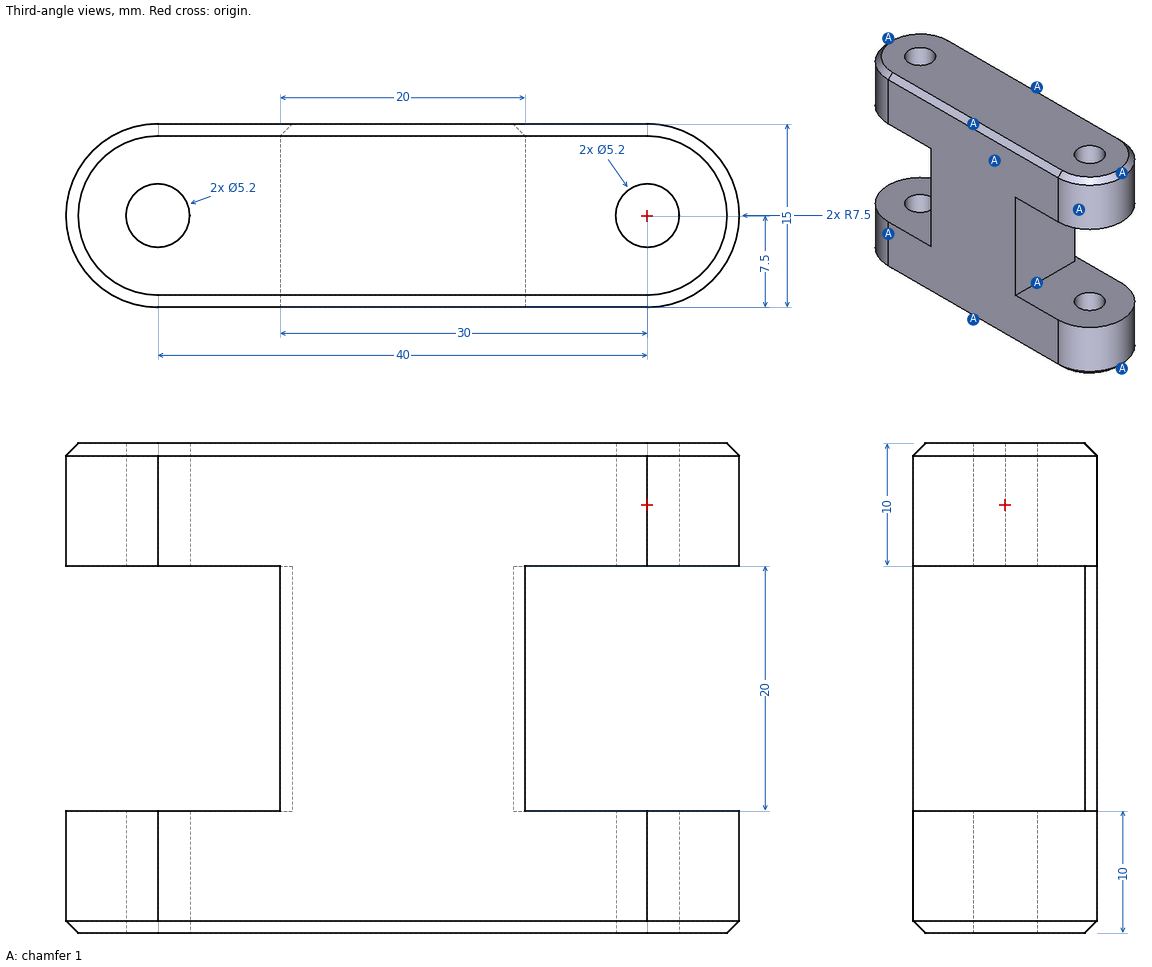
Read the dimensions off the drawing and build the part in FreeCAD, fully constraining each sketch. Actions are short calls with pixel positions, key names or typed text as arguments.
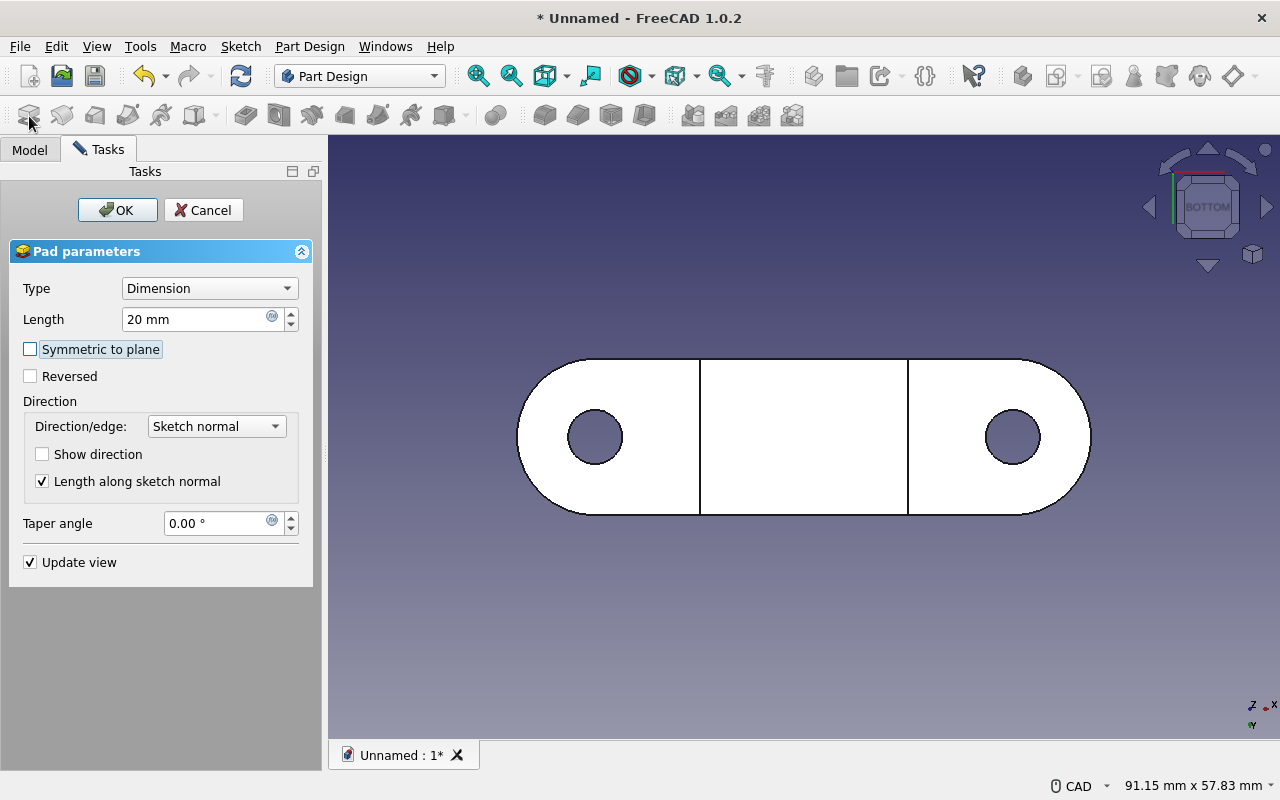
click(118, 210)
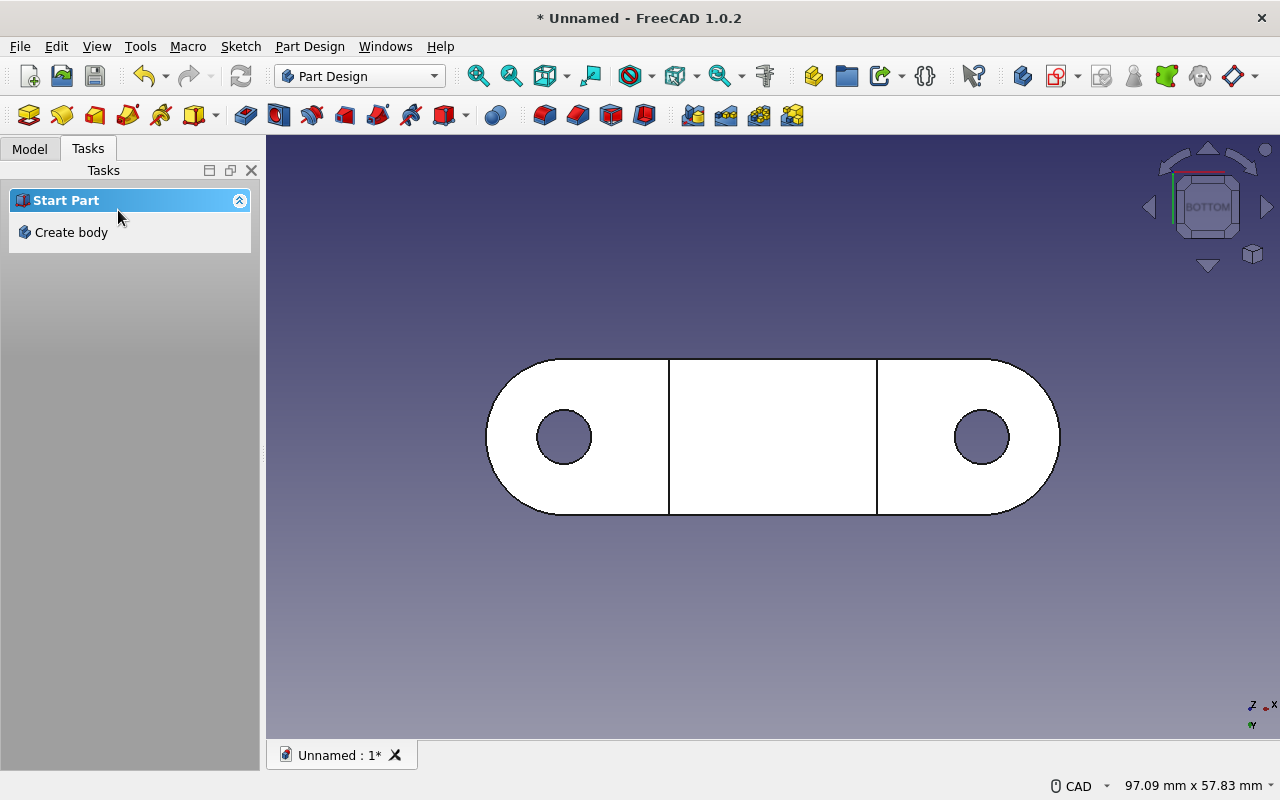
click(773, 436)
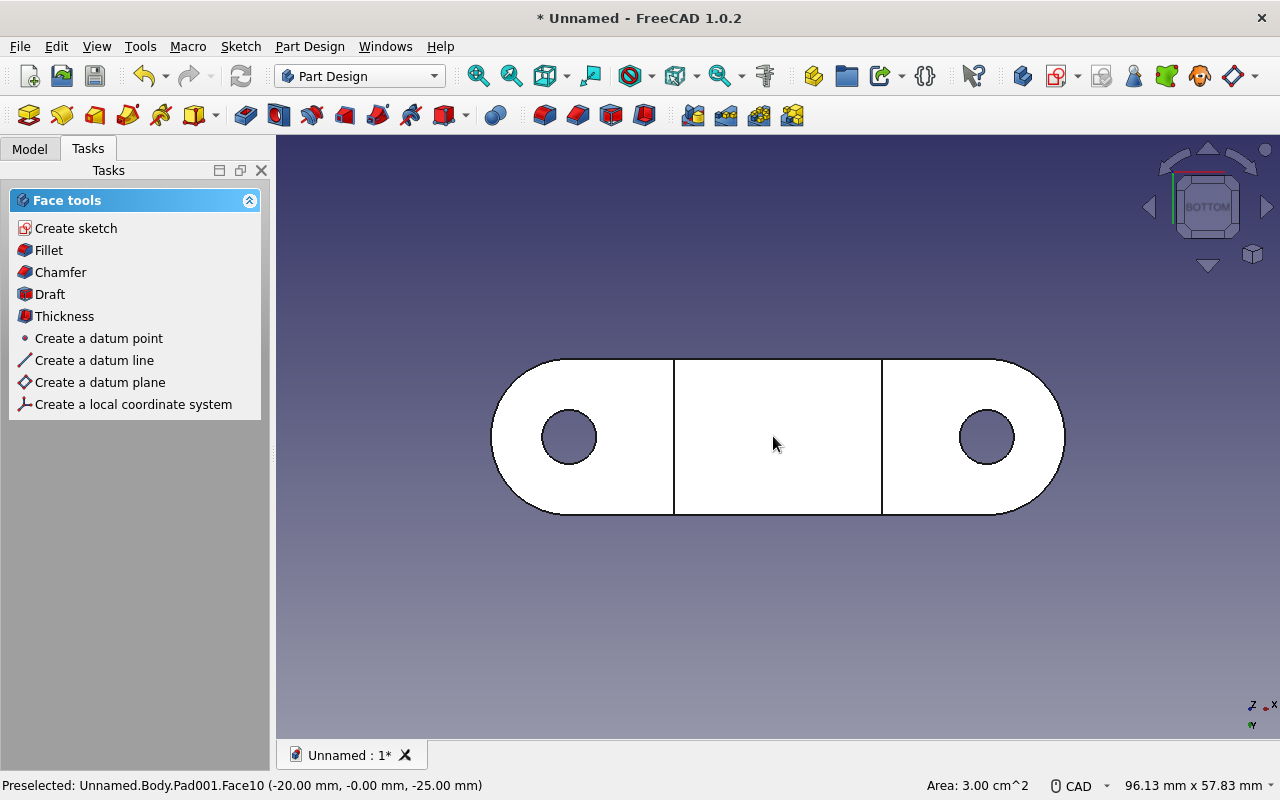
click(1056, 76)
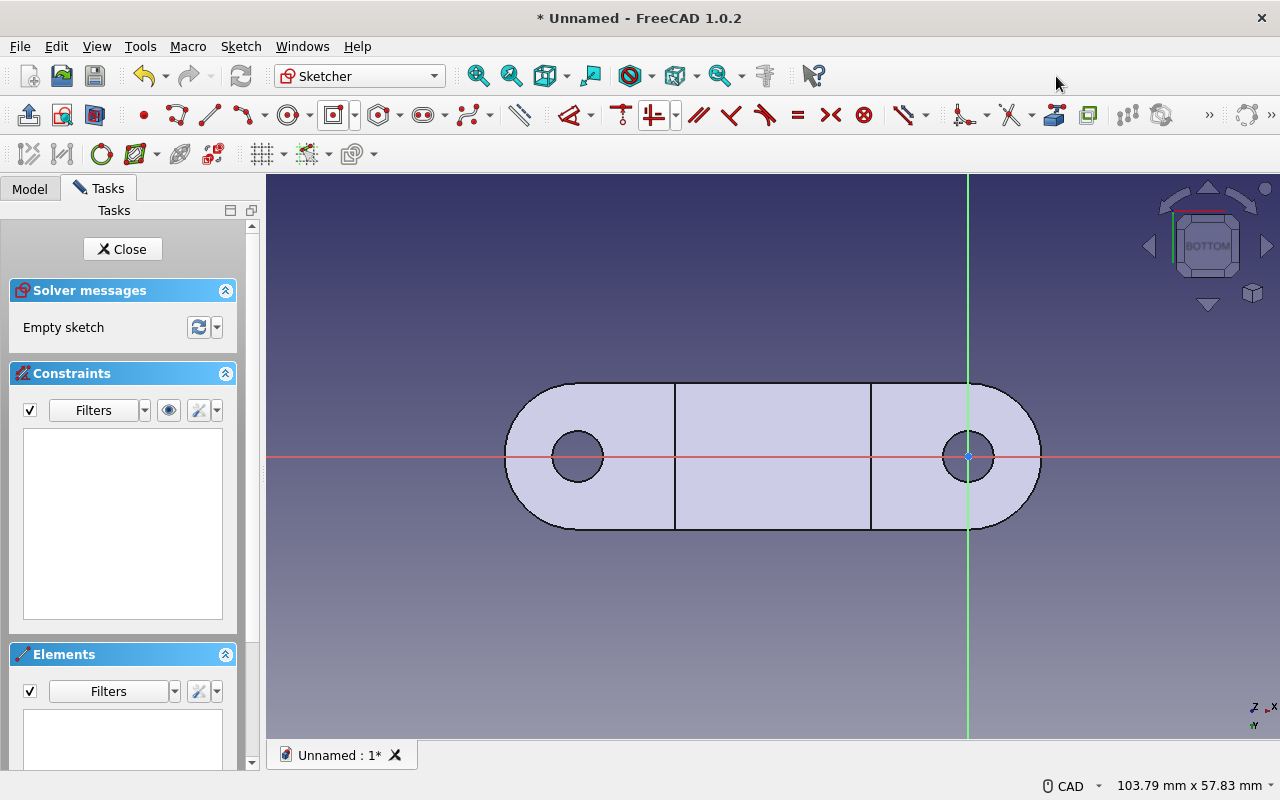
key(g)
key(s)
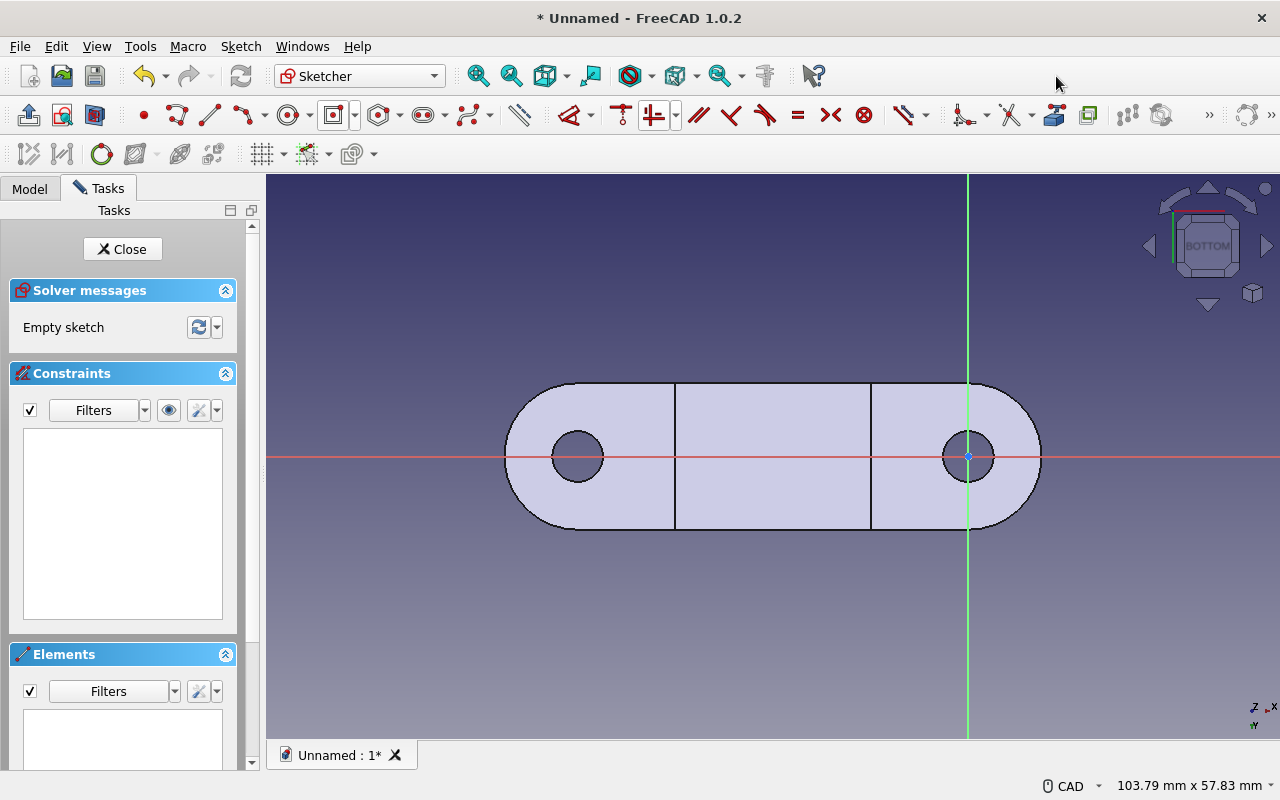
click(968, 457)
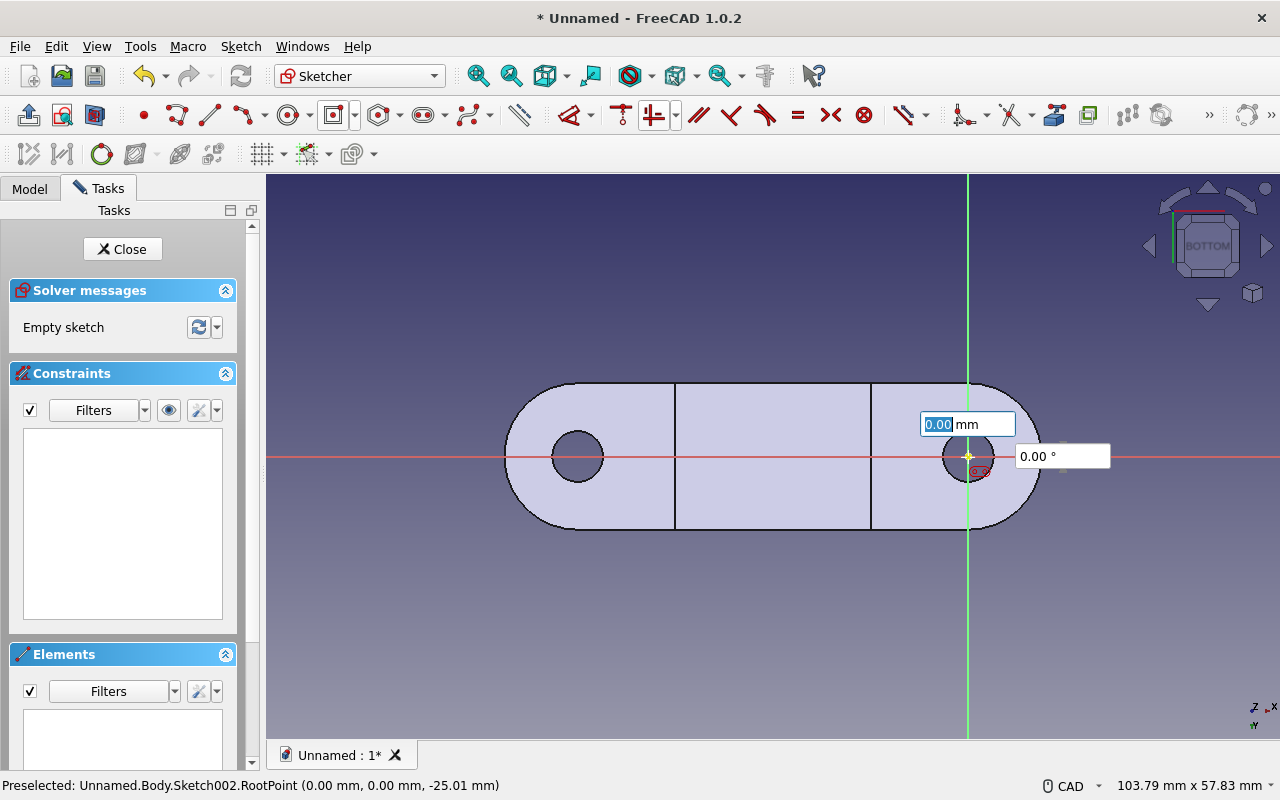
click(578, 448)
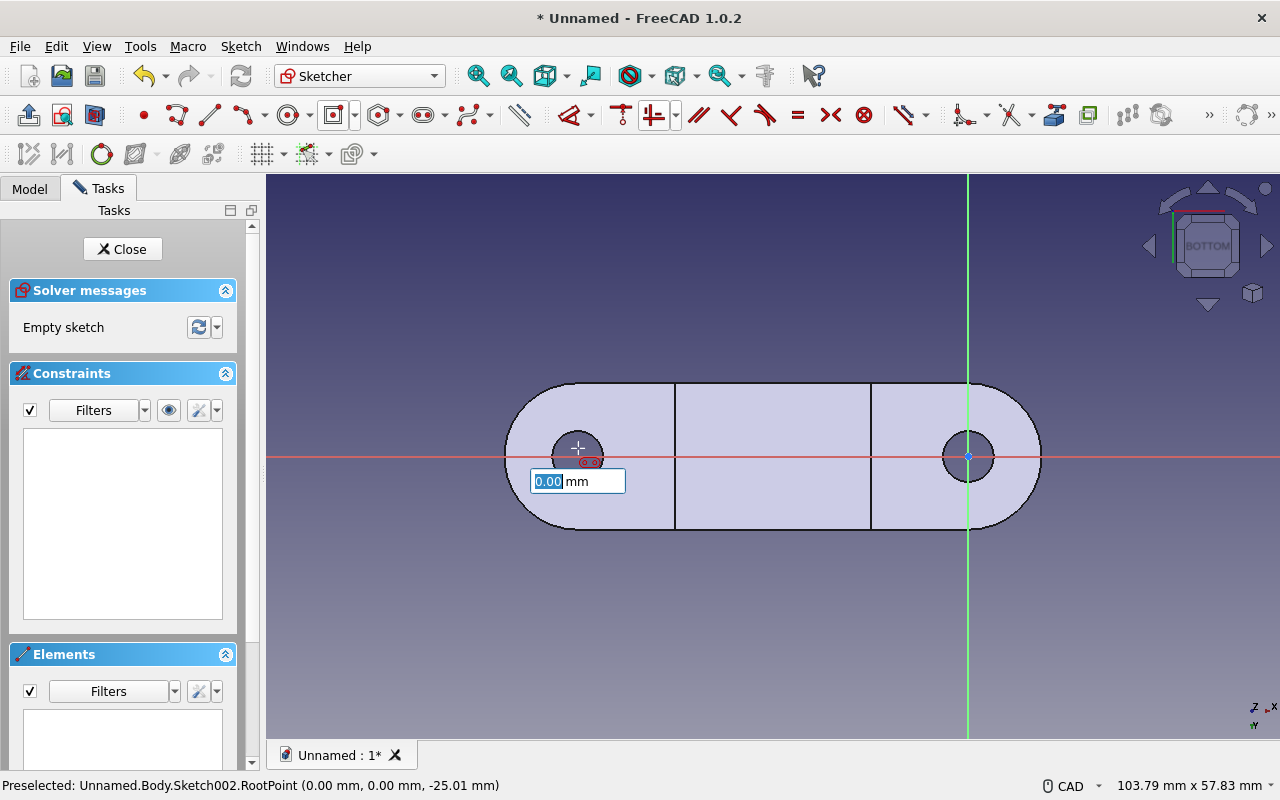
click(773, 530)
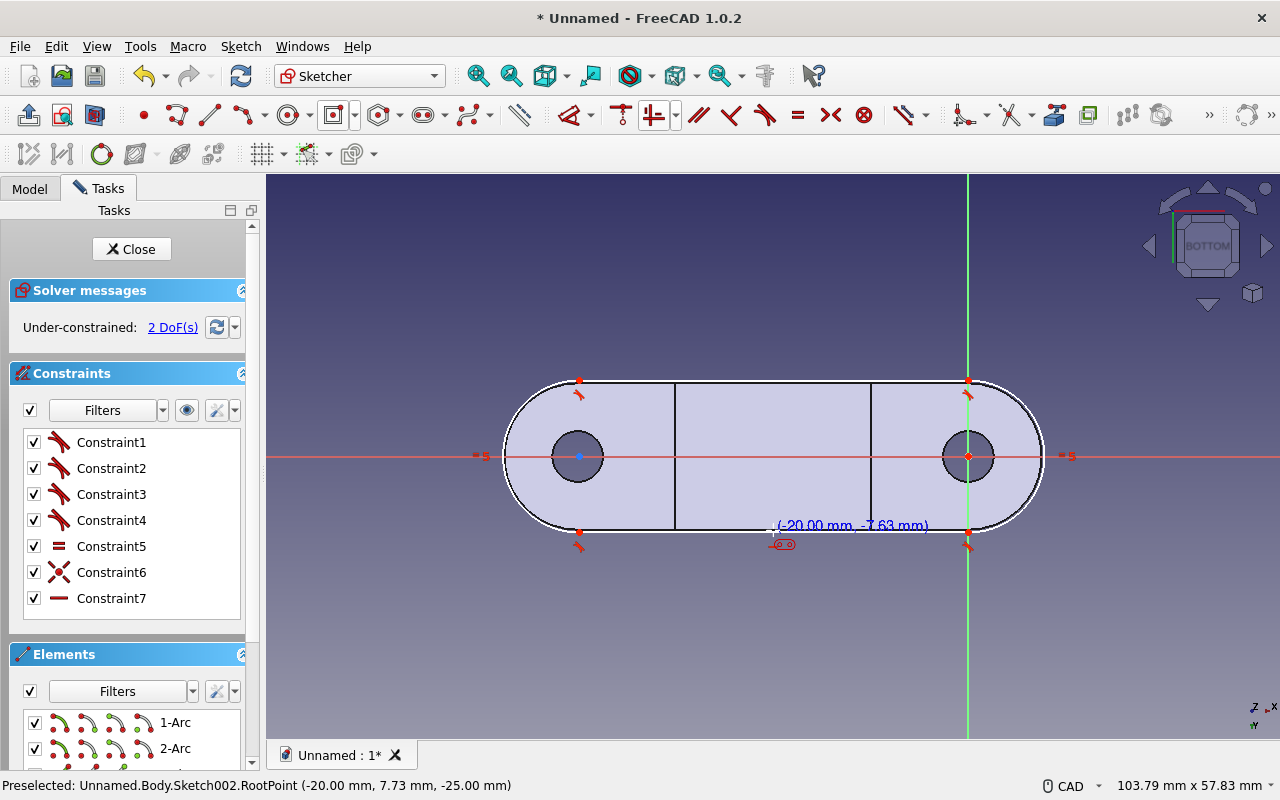
key(g)
key(c)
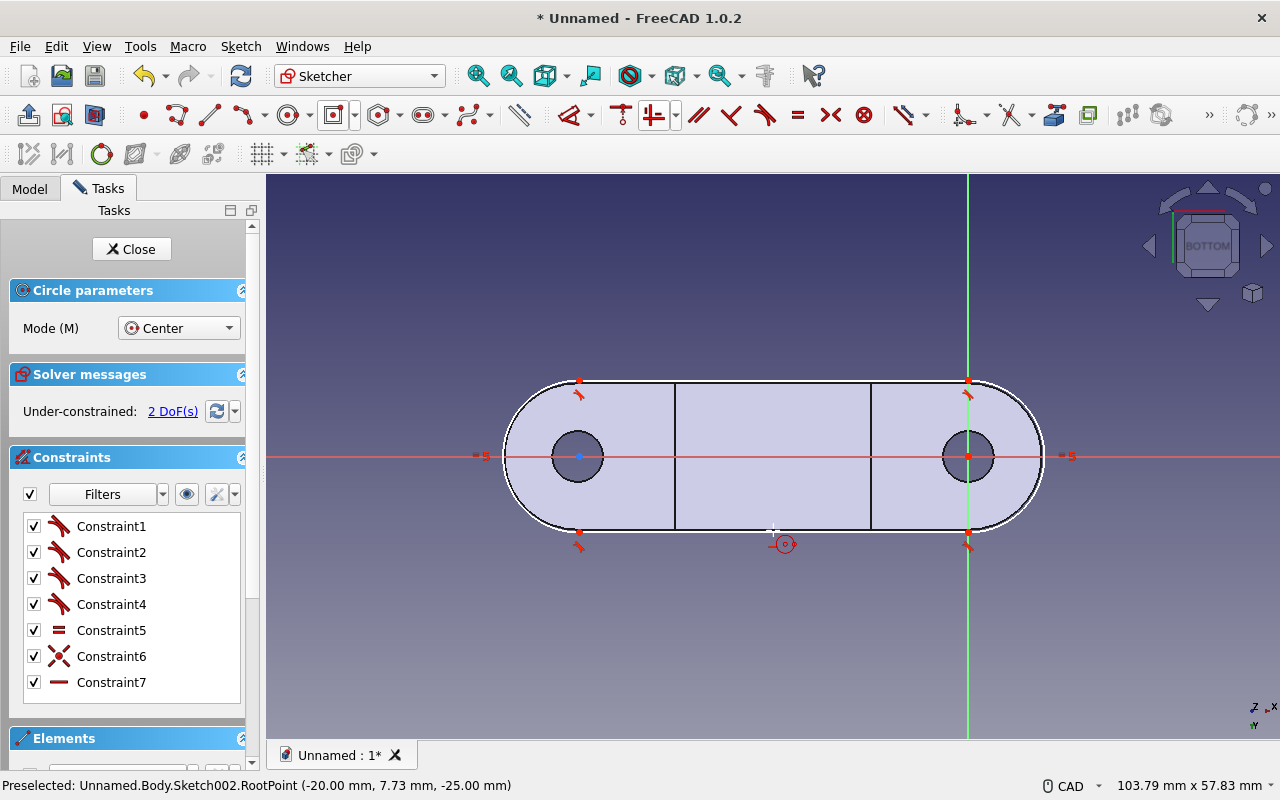
click(579, 457)
move(596, 439)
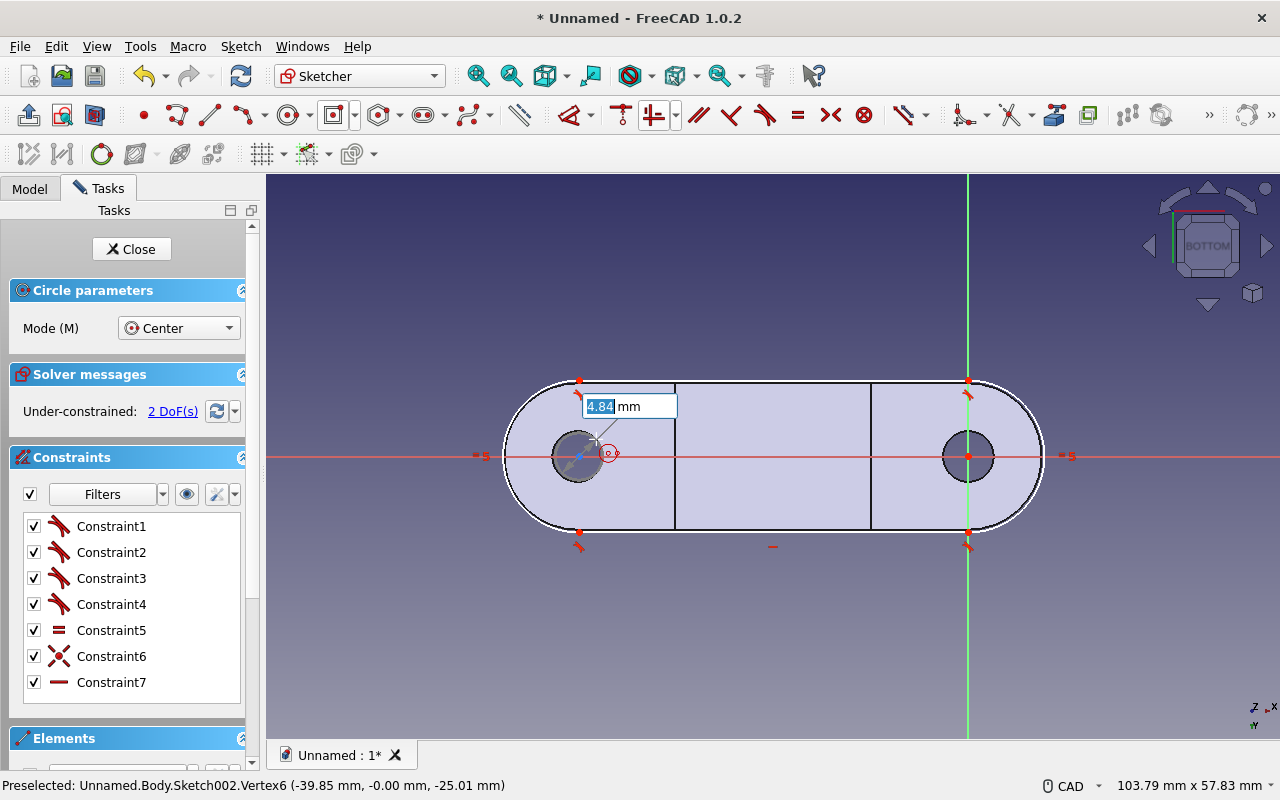
text(5.2)
key(Return)